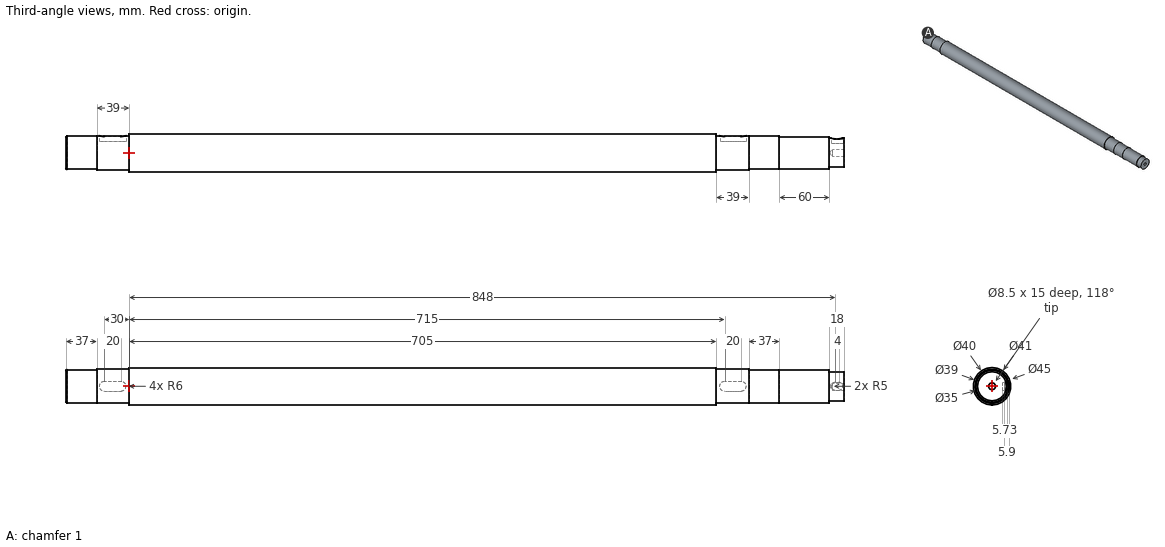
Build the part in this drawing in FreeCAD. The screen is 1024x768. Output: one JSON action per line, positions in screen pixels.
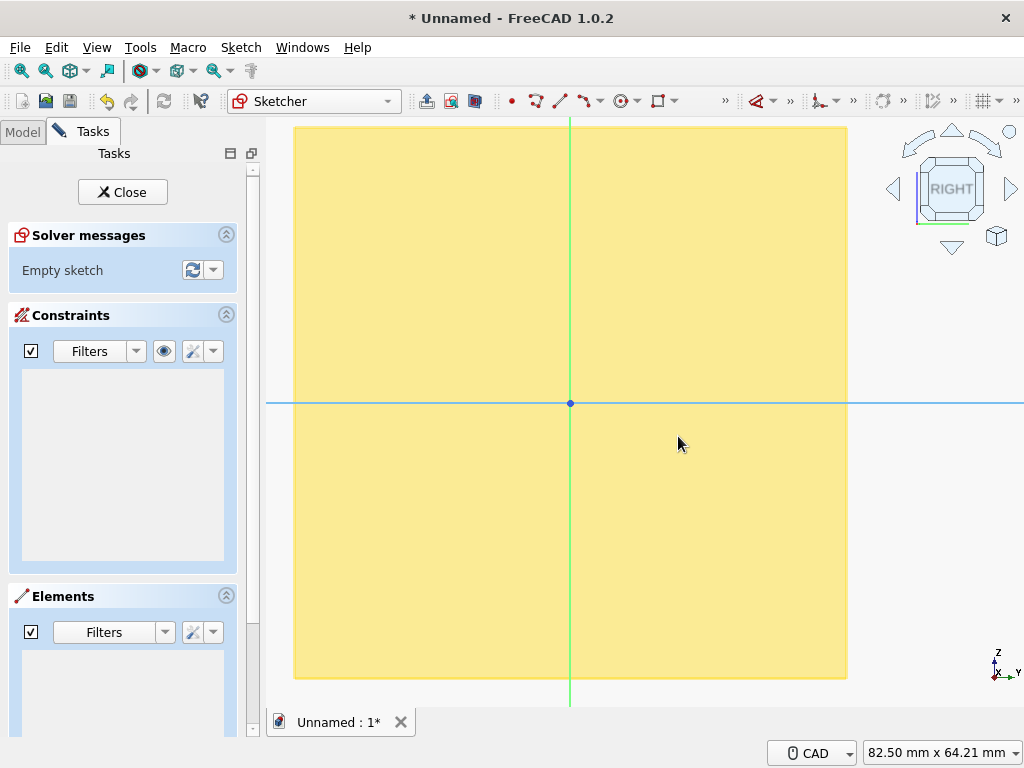
{"action": "left_click", "coordinate": [622, 102]}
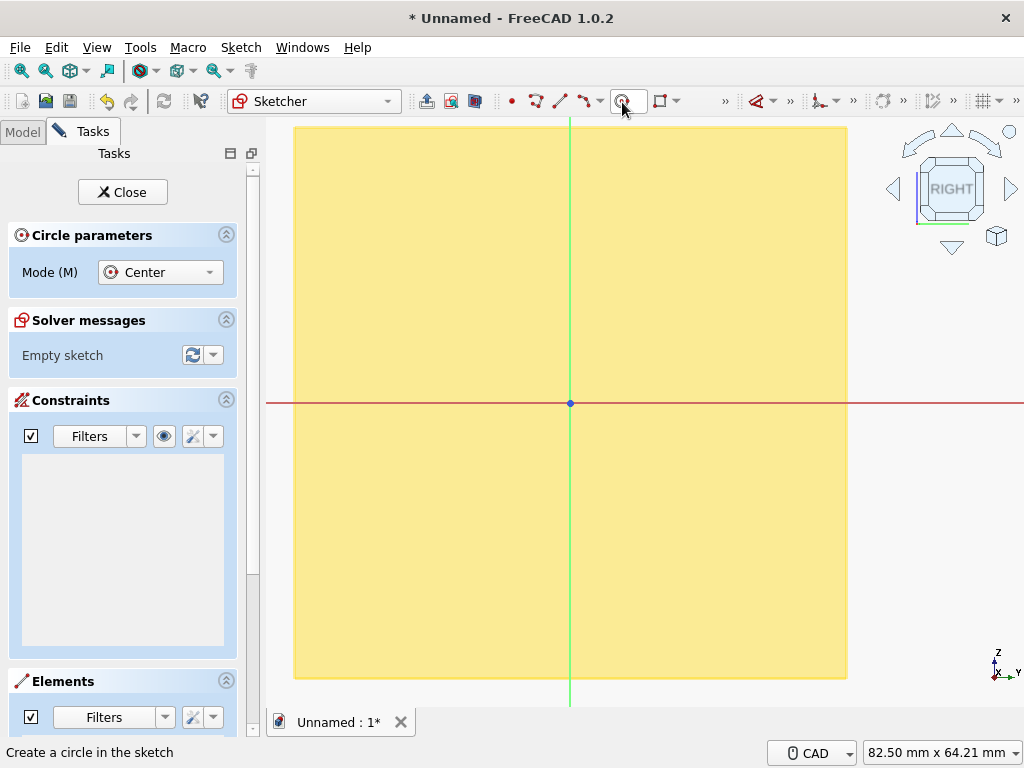
{"action": "left_click", "coordinate": [570, 403]}
{"action": "mouse_move", "coordinate": [704, 270]}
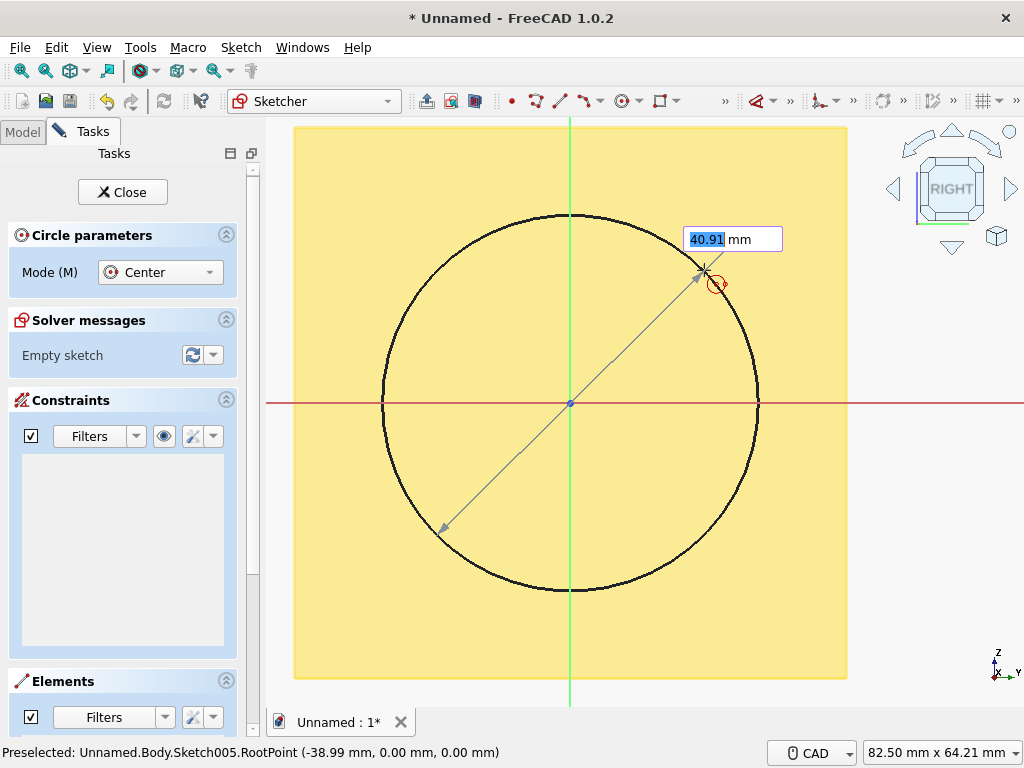
{"action": "type", "text": "41"}
{"action": "key", "text": "Return"}
{"action": "key", "text": "Escape"}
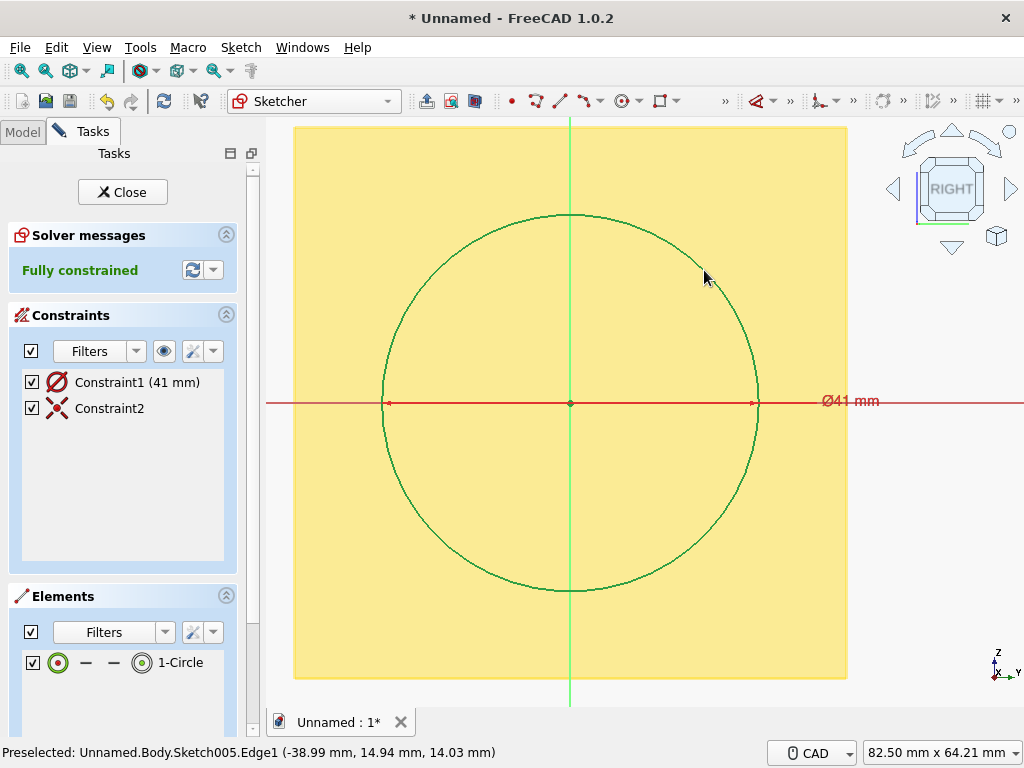
{"action": "left_click", "coordinate": [123, 192]}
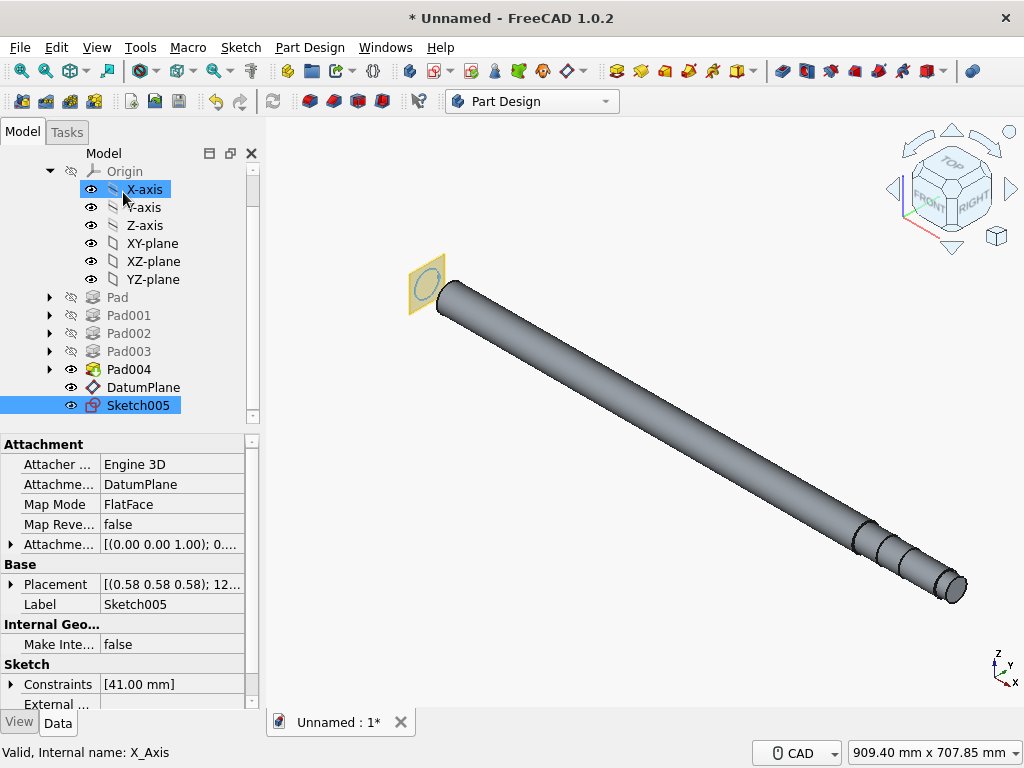
{"action": "left_click", "coordinate": [618, 72]}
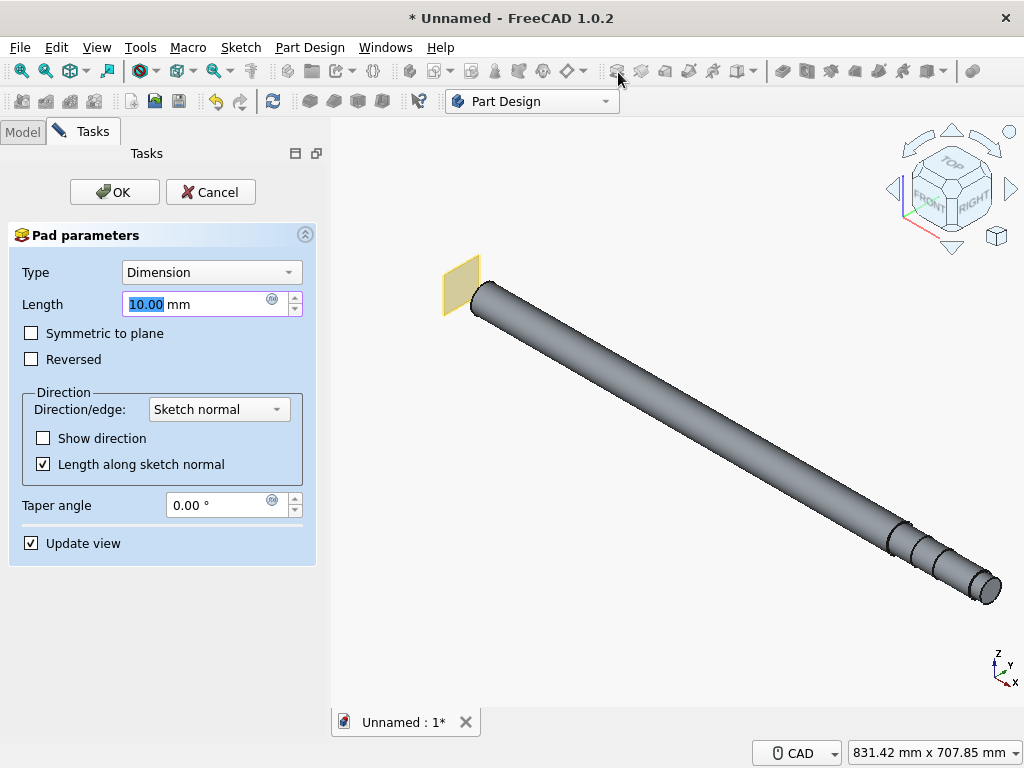
{"action": "type", "text": "39"}
{"action": "key", "text": "Tab"}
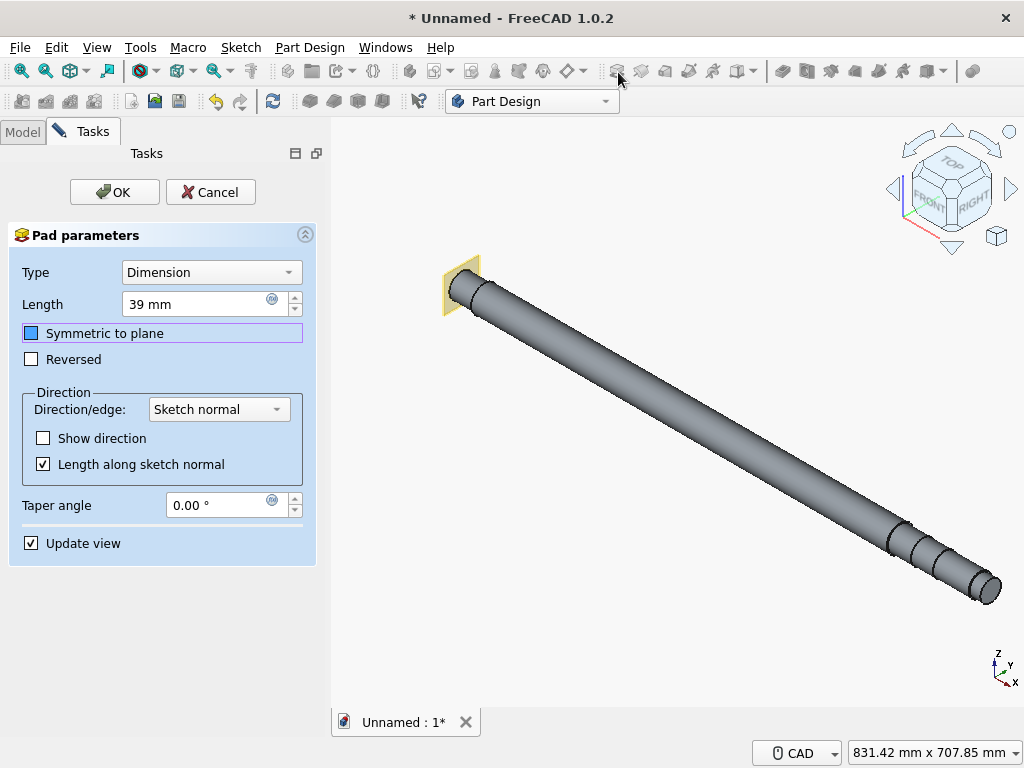
{"action": "left_click", "coordinate": [115, 192]}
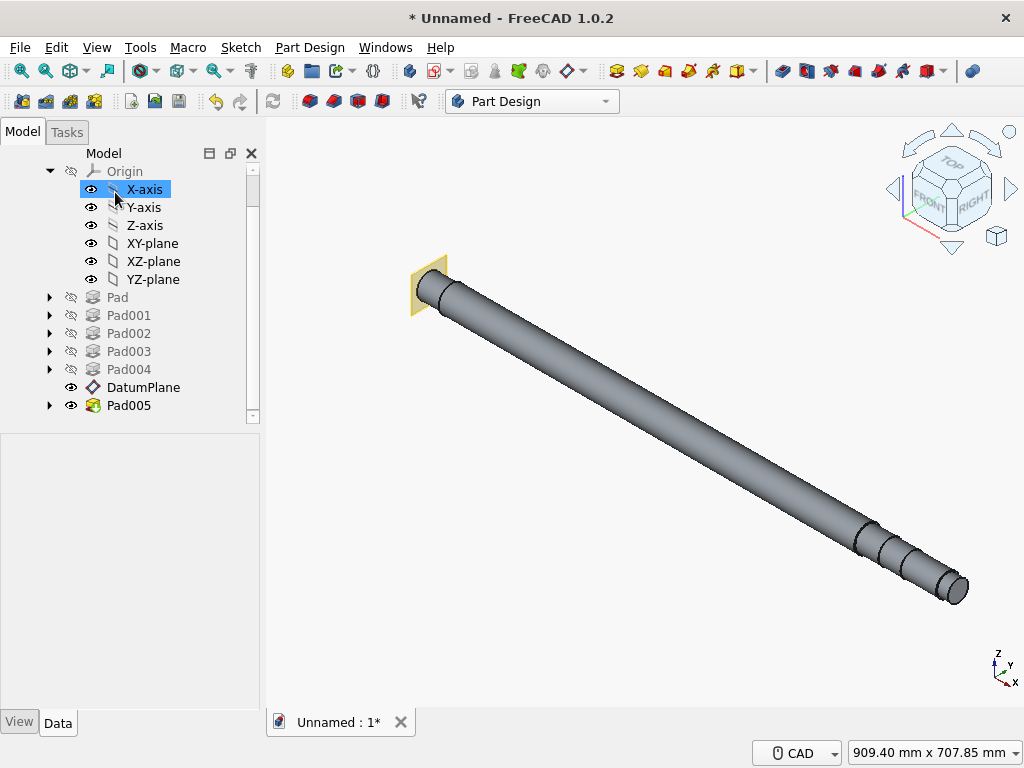
{"action": "left_click", "coordinate": [116, 387]}
{"action": "key", "text": "space"}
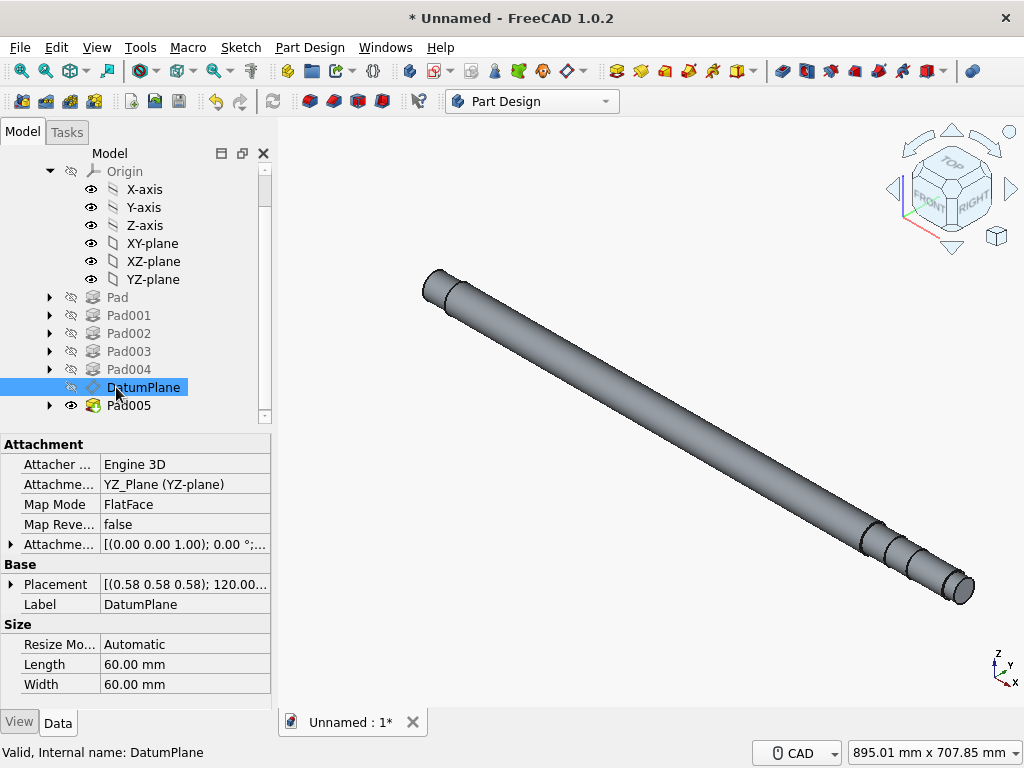
{"action": "left_click", "coordinate": [136, 279]}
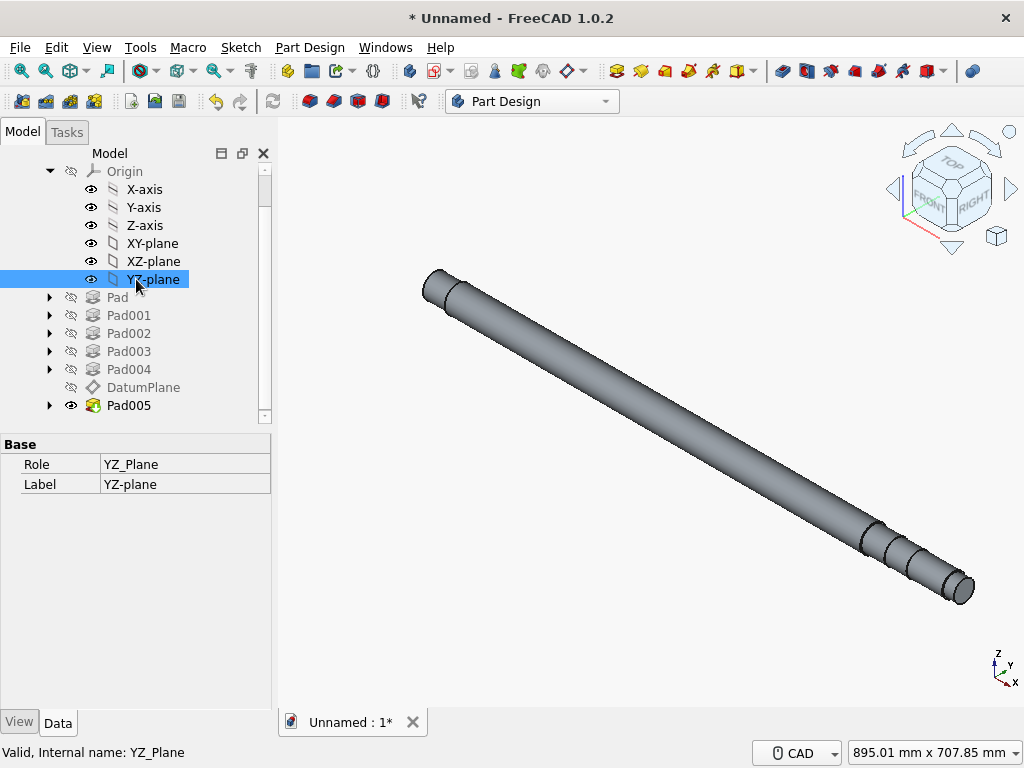
{"action": "left_click", "coordinate": [568, 72]}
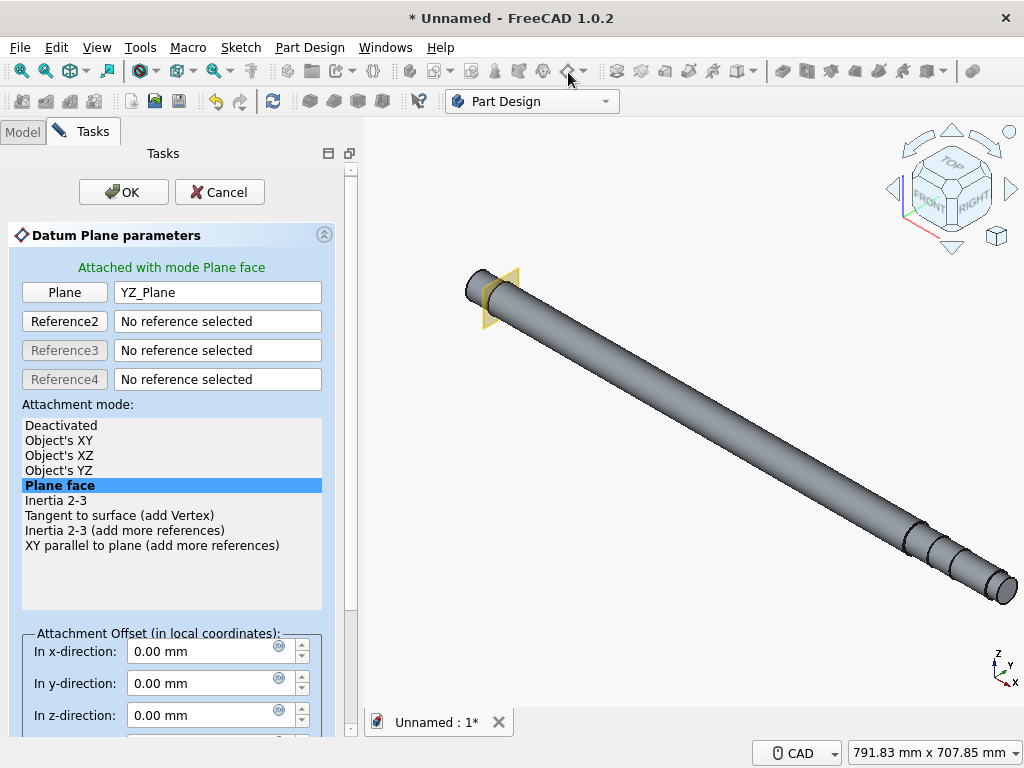
{"action": "triple_click", "coordinate": [210, 715]}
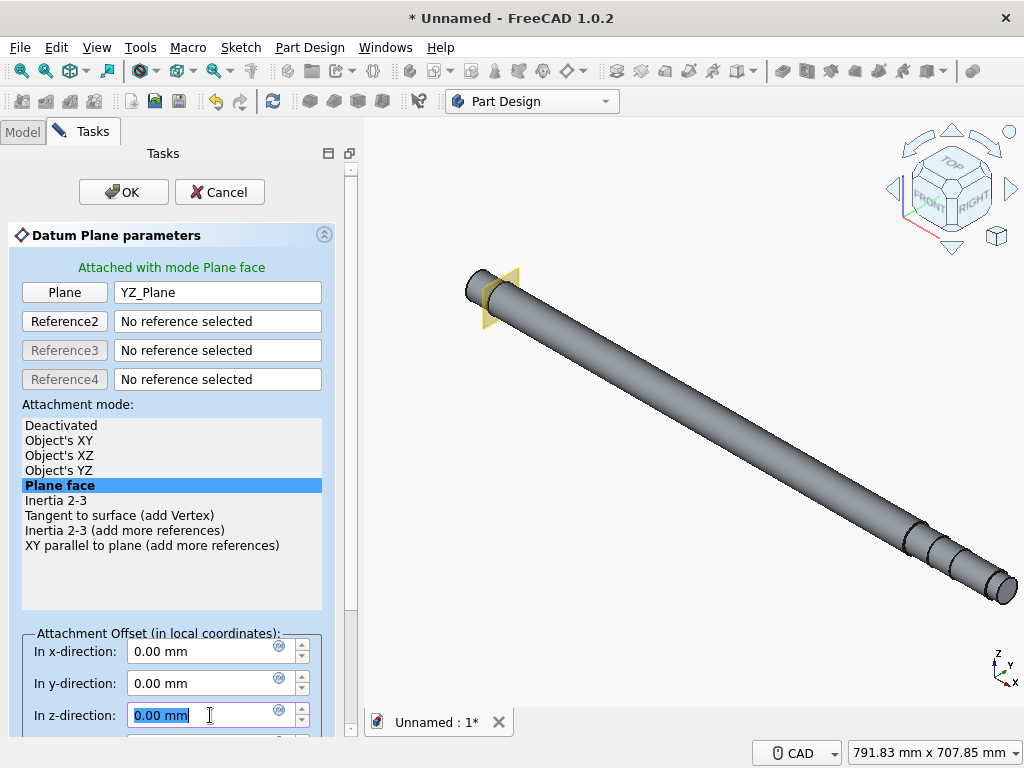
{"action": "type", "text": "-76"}
{"action": "key", "text": "Tab"}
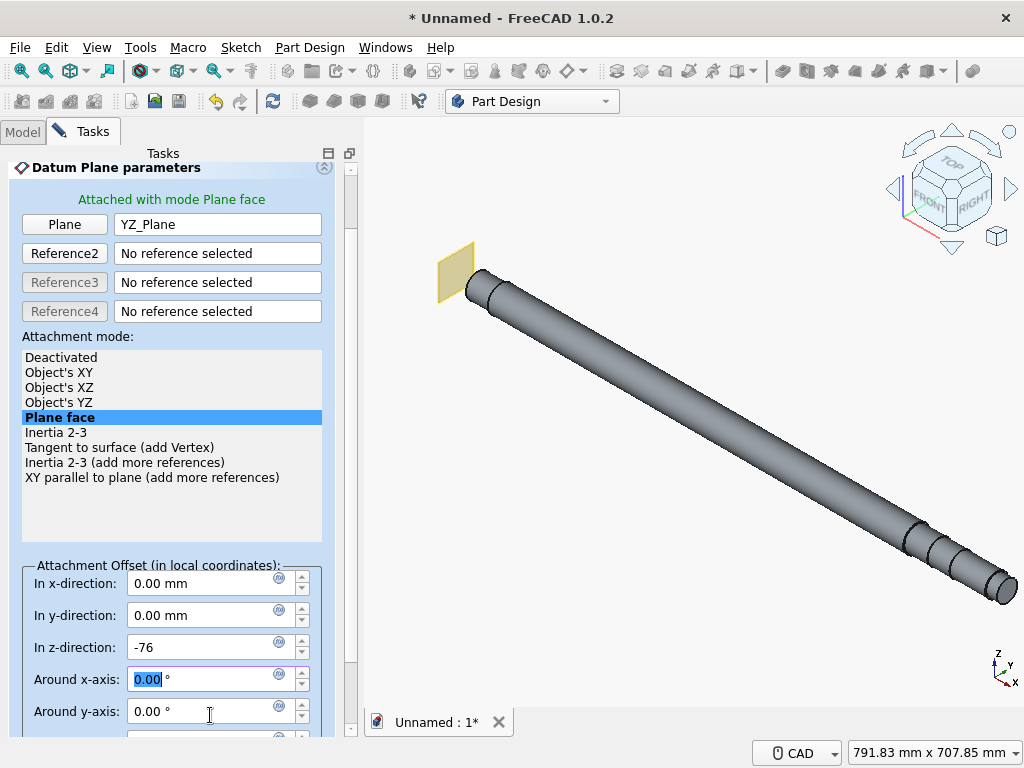
{"action": "scroll", "coordinate": [351, 450], "scroll_direction": "up", "scroll_amount": 2}